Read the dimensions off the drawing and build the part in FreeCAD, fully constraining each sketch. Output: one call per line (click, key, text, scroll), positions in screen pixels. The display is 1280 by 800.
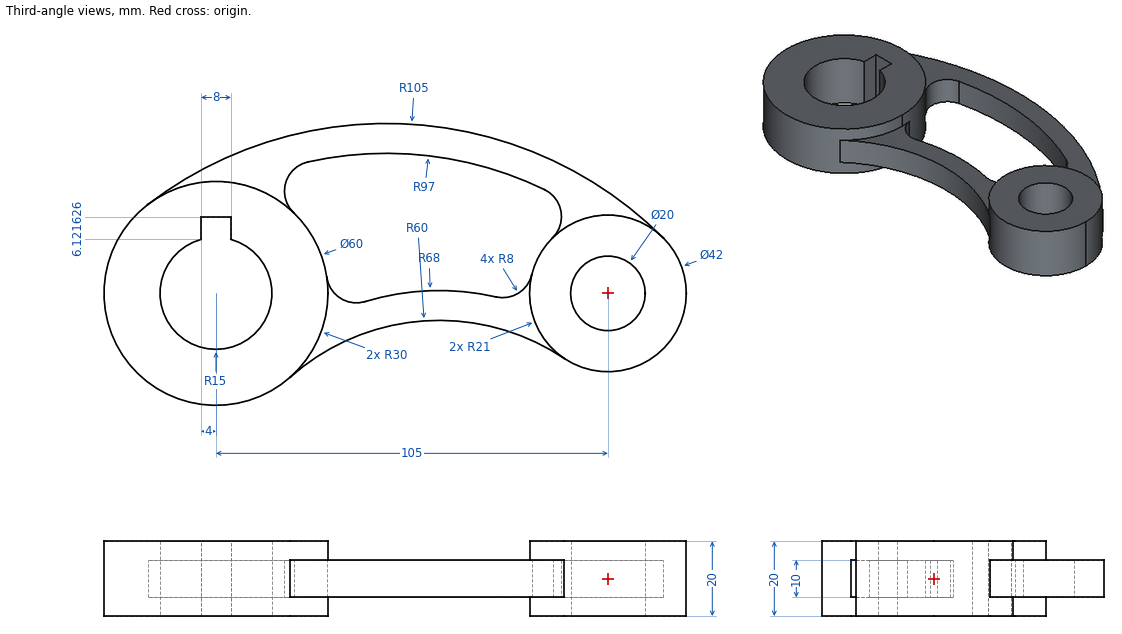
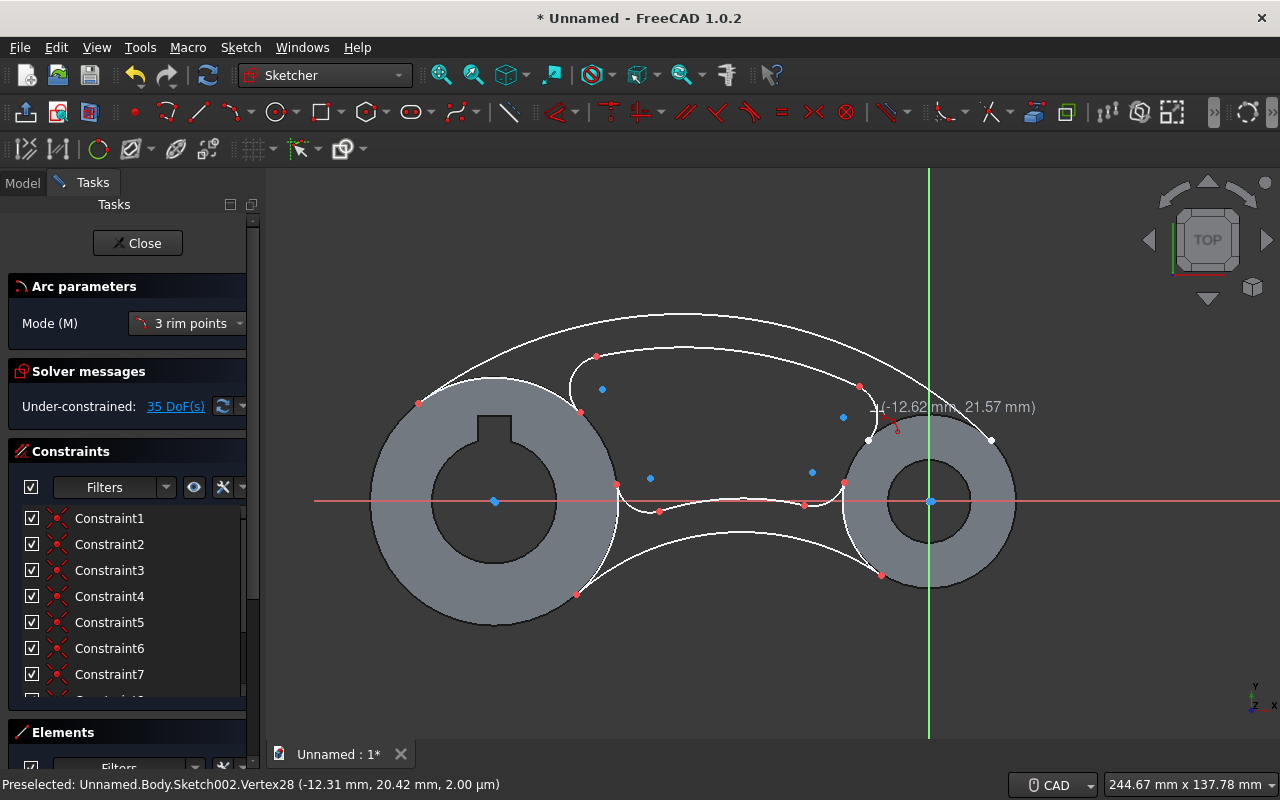
click(868, 441)
click(991, 441)
click(903, 419)
key(Escape)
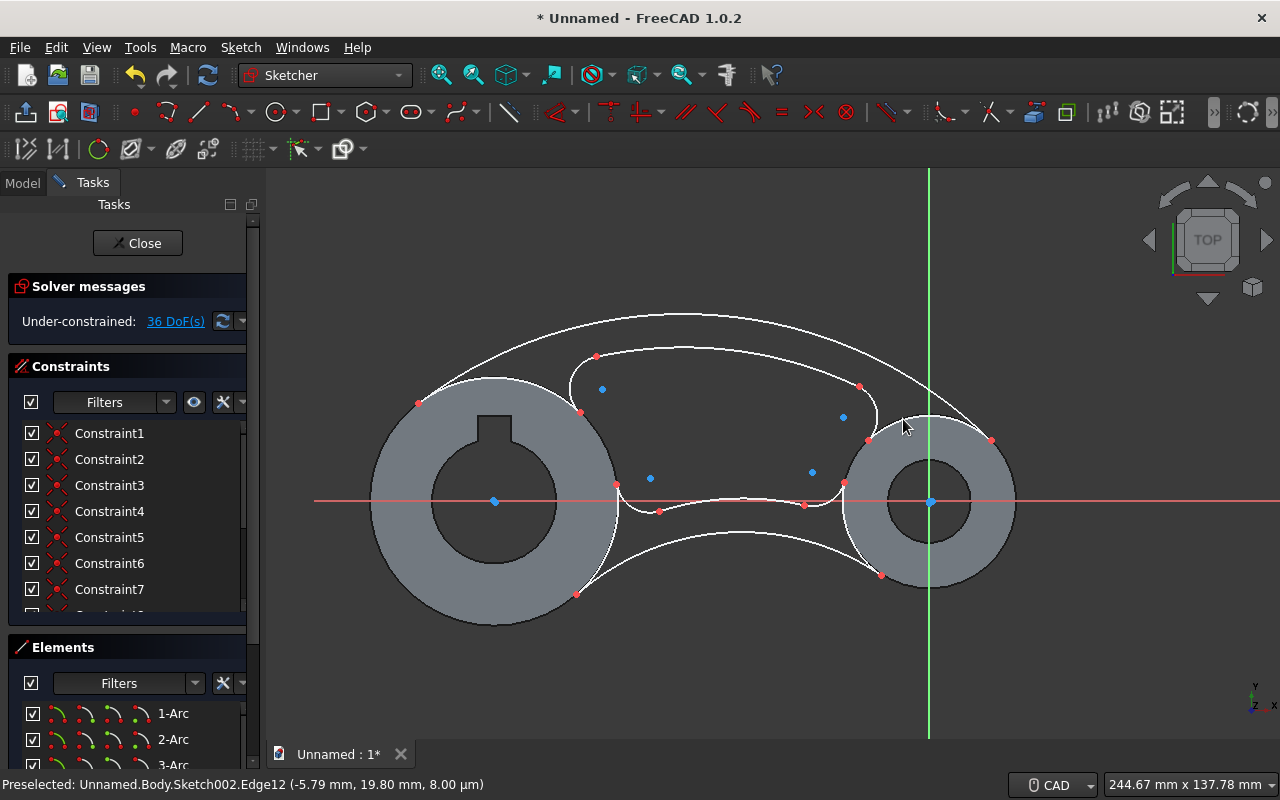
click(843, 514)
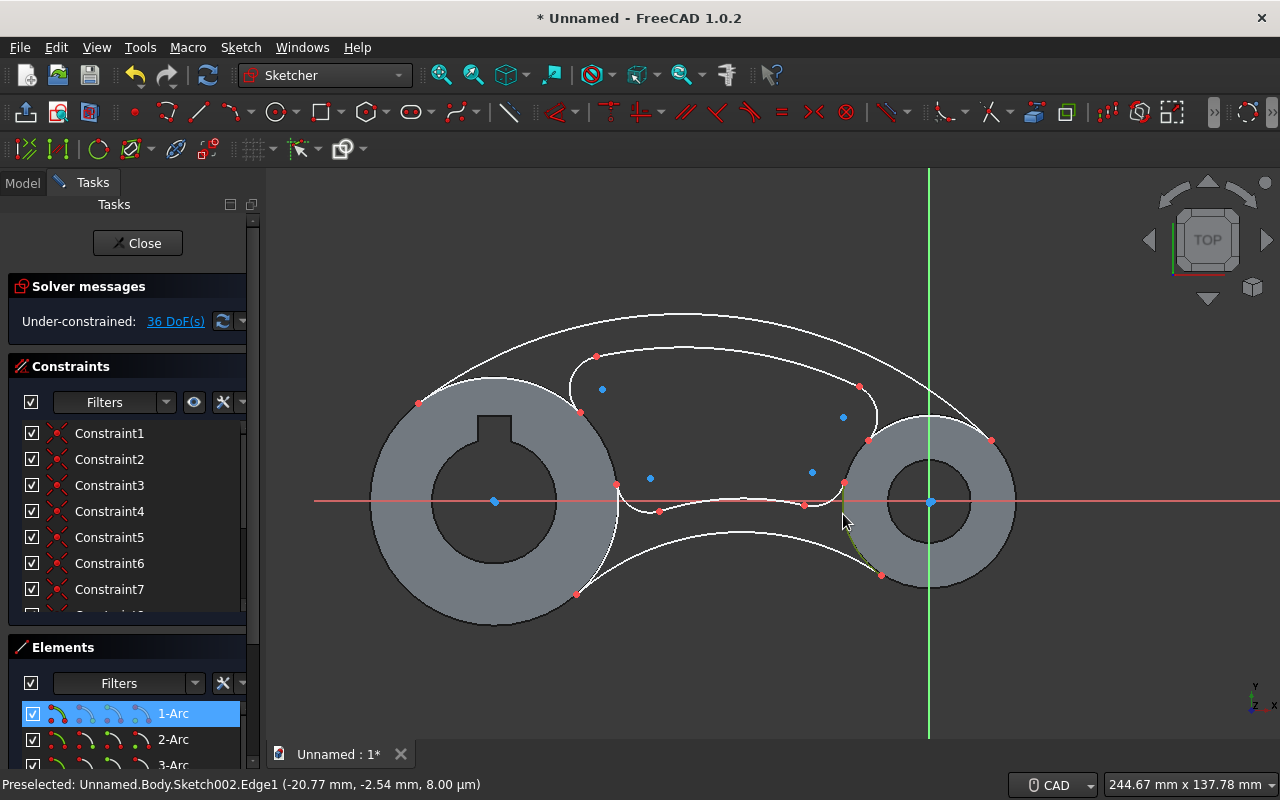
click(829, 502)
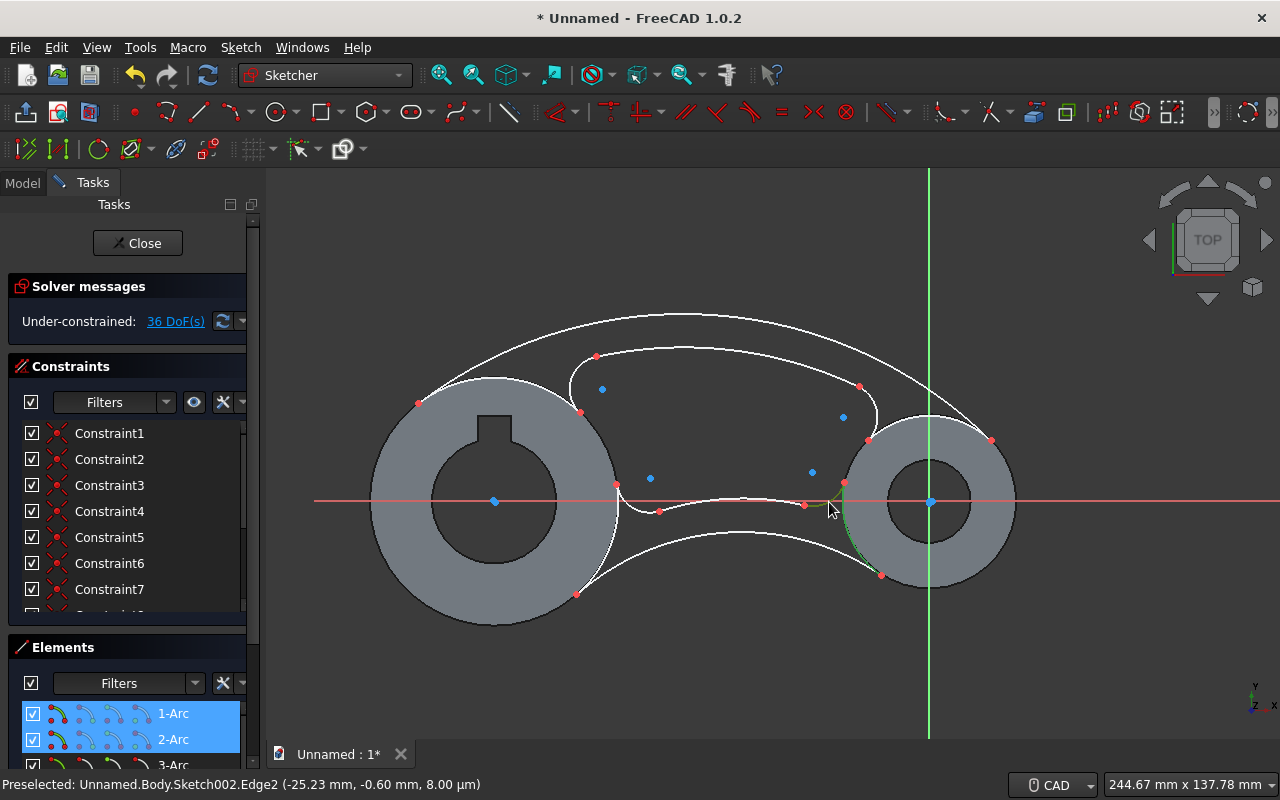
key(t)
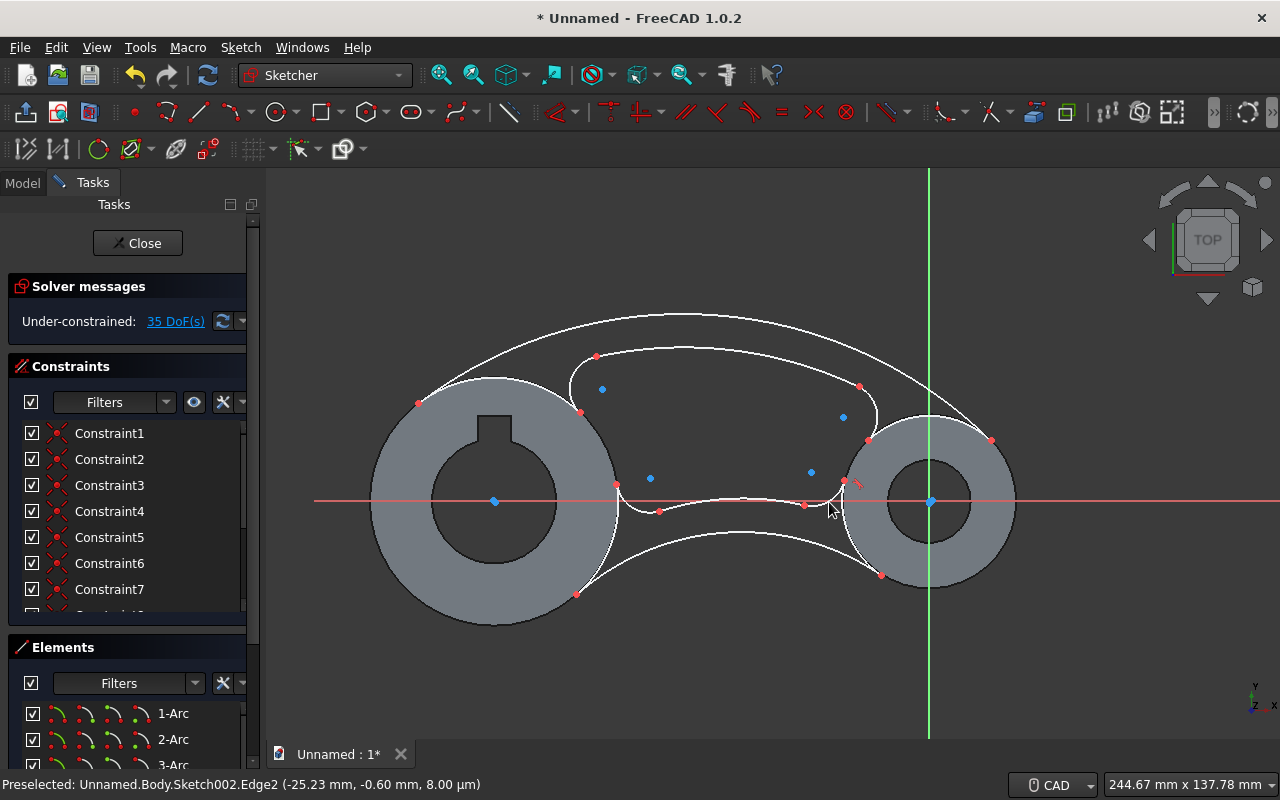
scroll(843, 512, up, 2)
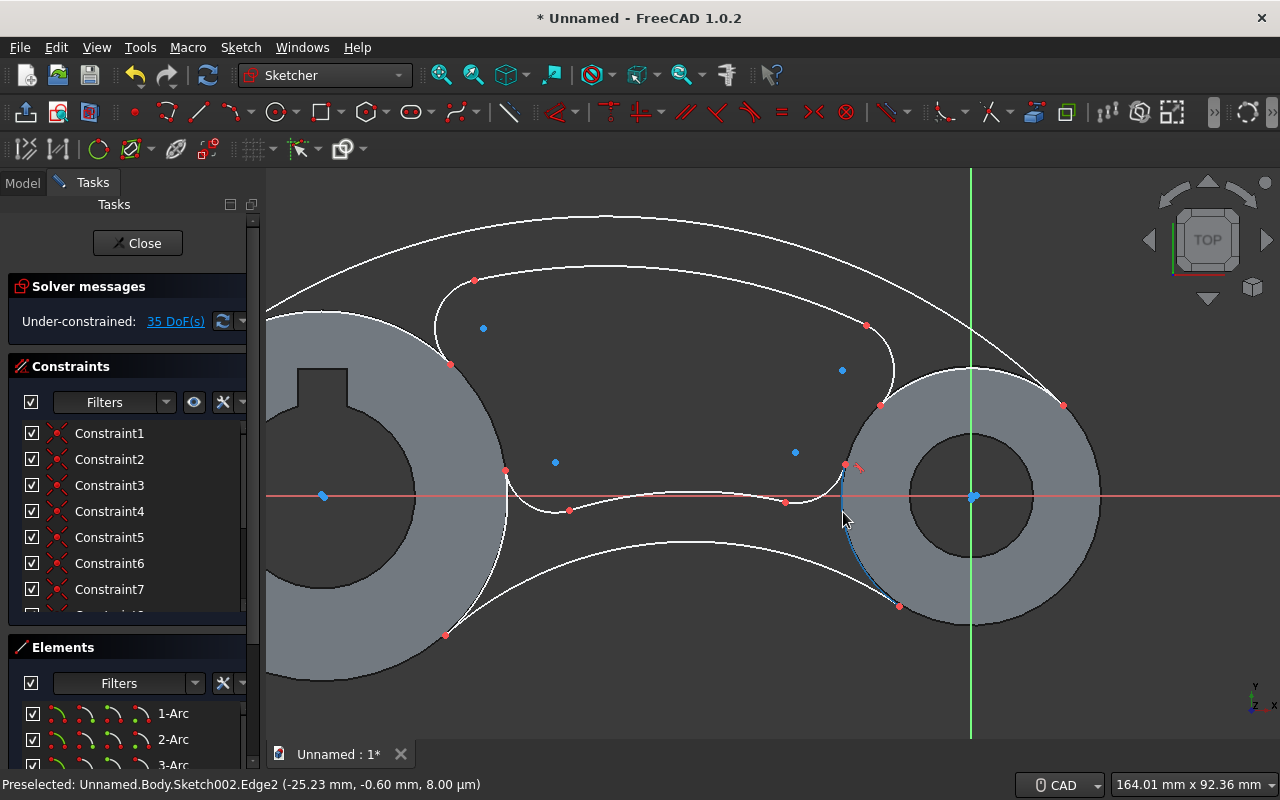
click(843, 512)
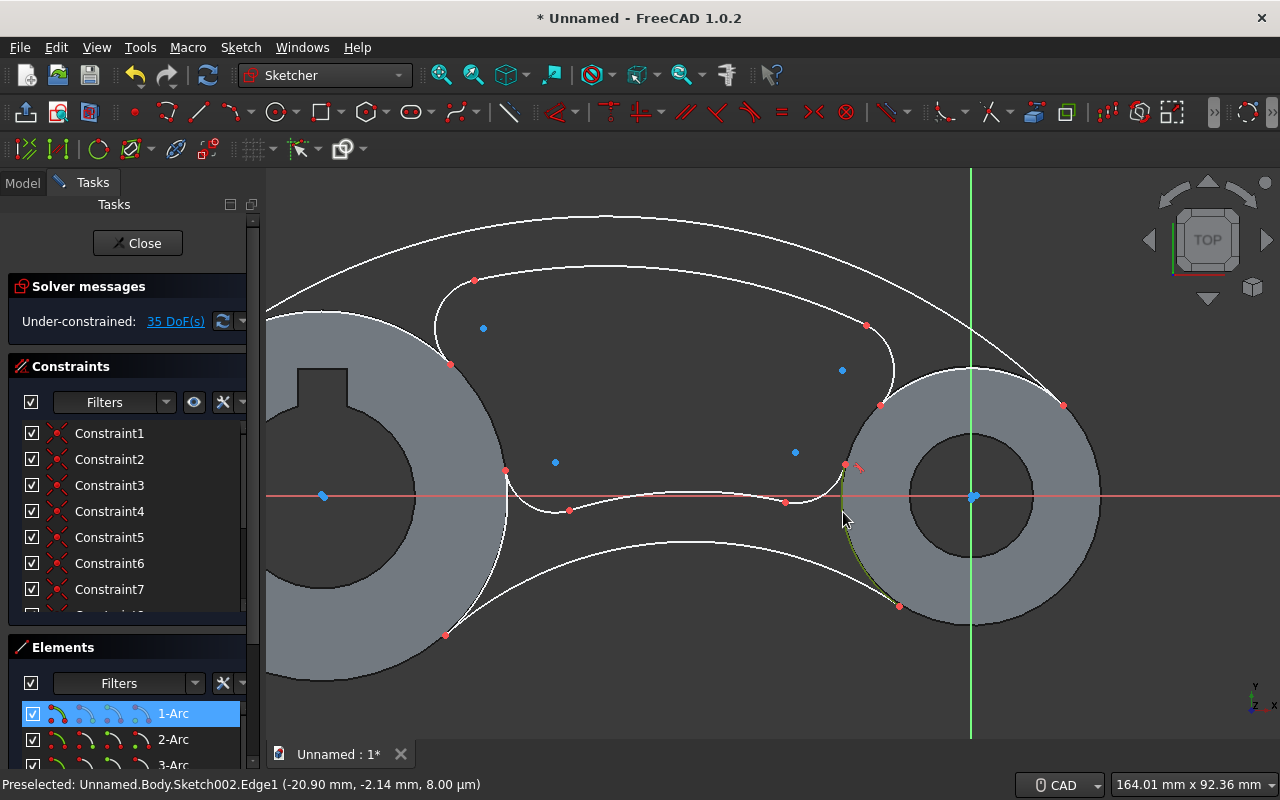
click(765, 549)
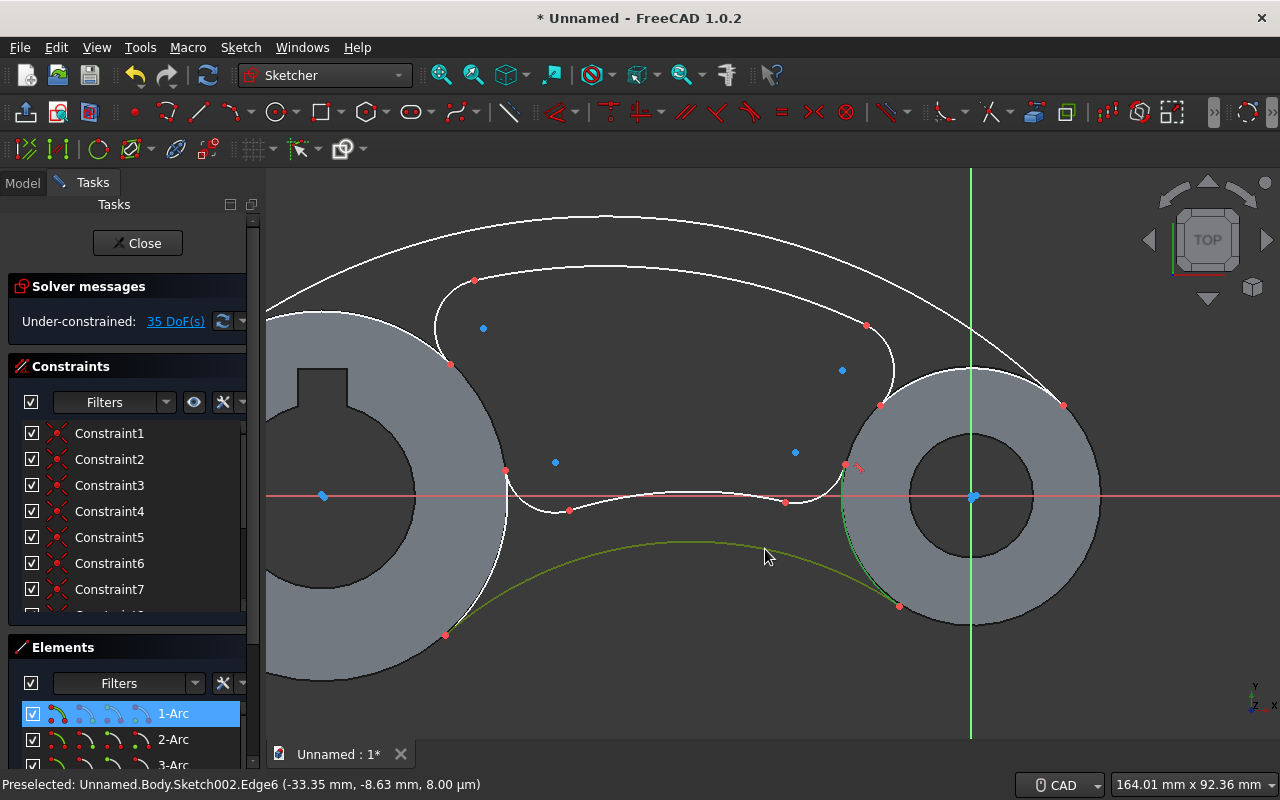
click(750, 112)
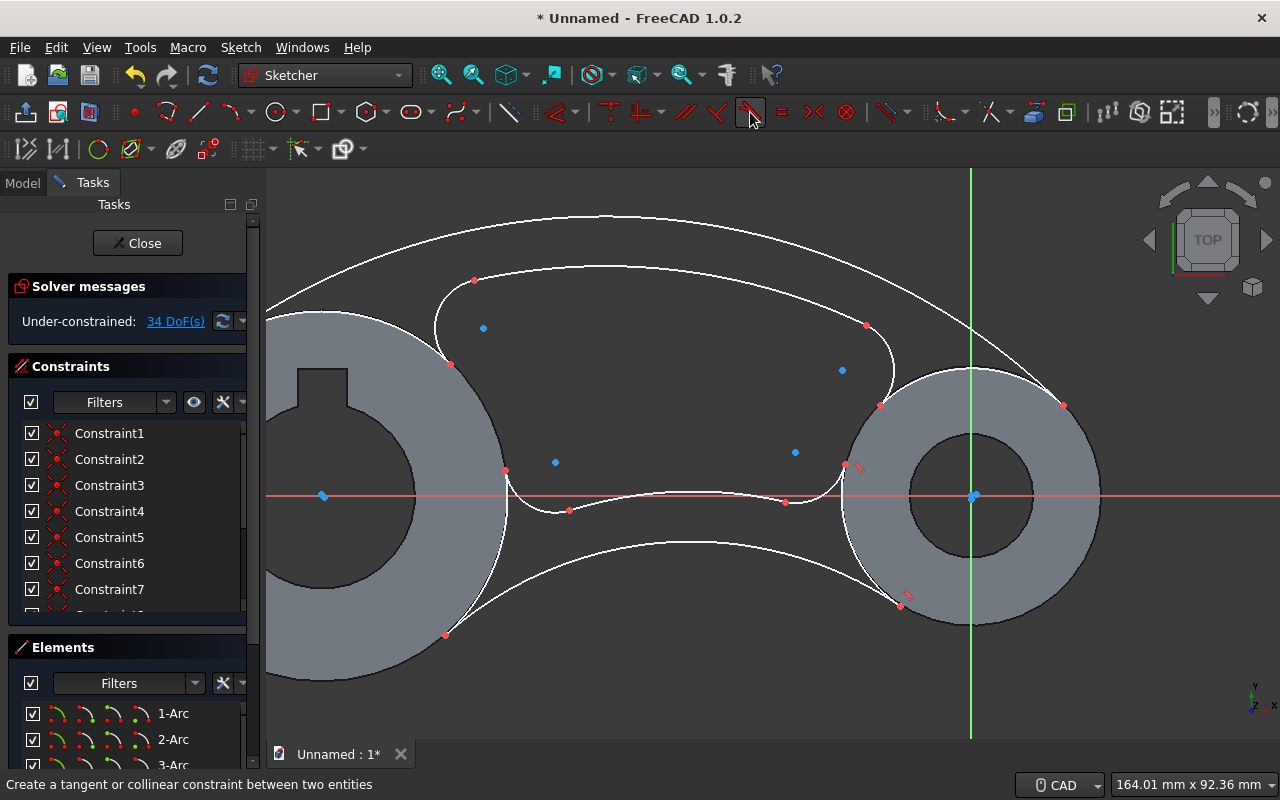
click(823, 495)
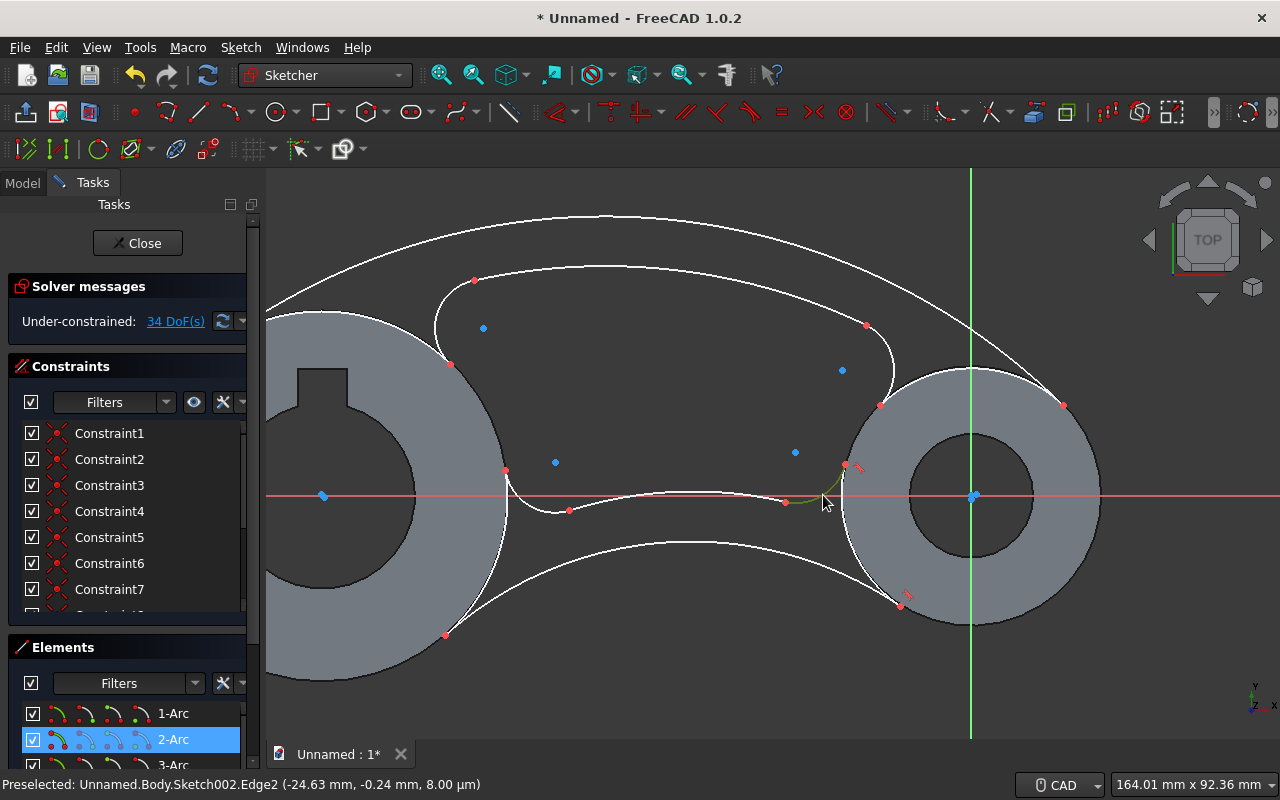
click(721, 492)